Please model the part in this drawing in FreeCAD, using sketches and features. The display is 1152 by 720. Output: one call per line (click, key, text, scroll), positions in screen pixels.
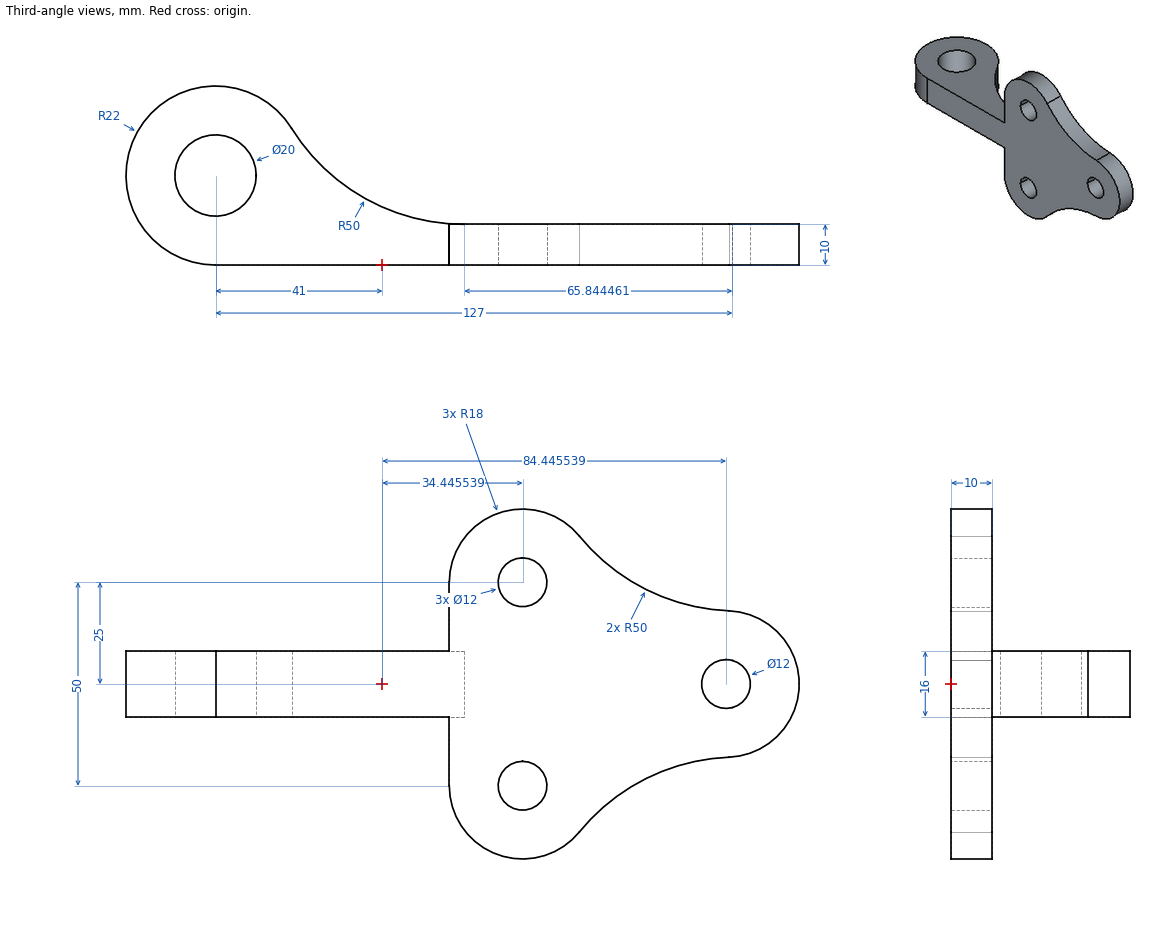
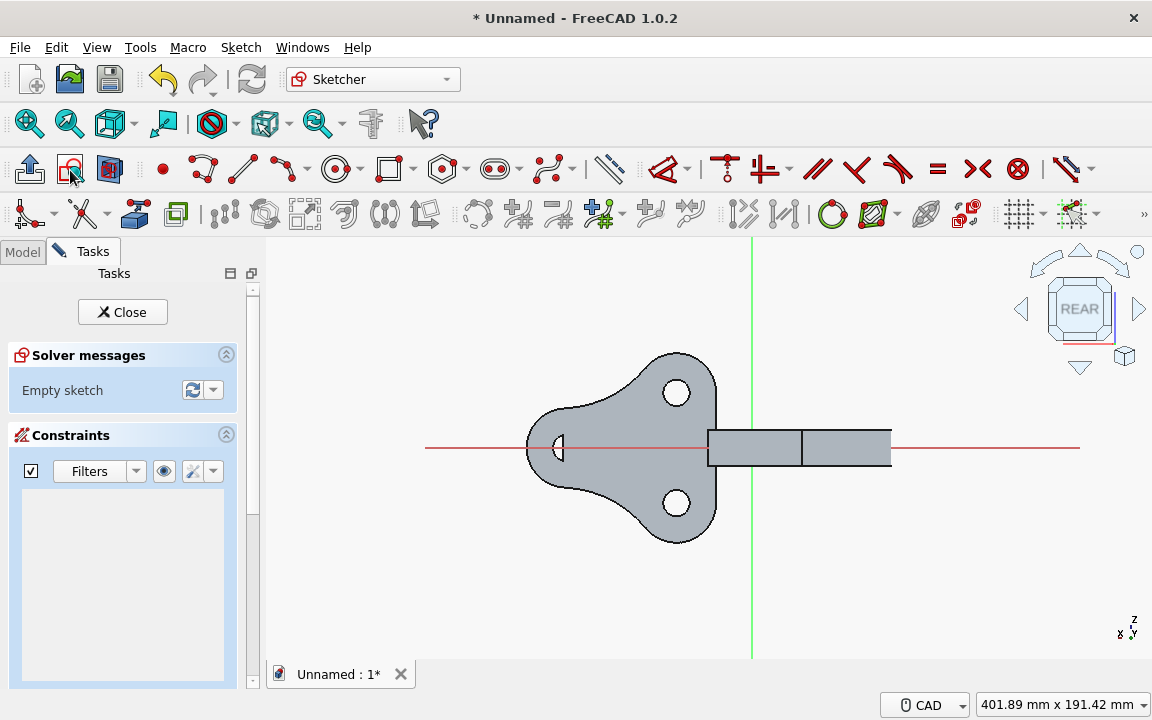
scroll(557, 448, up, 11)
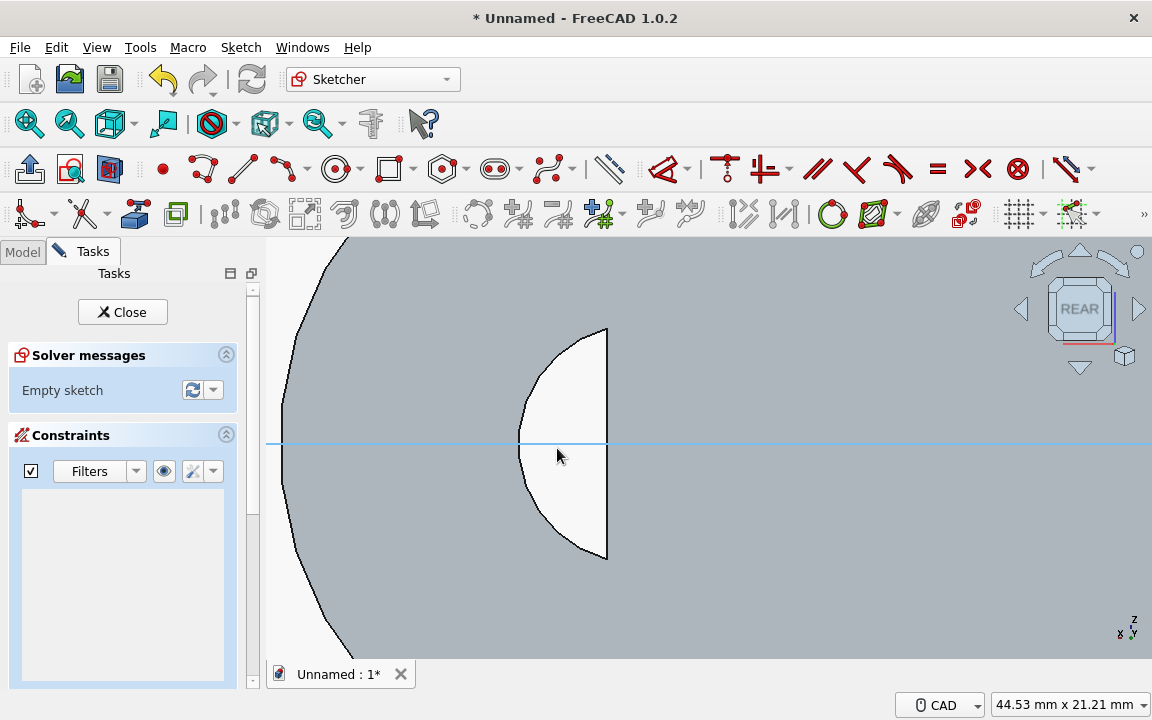
click(336, 170)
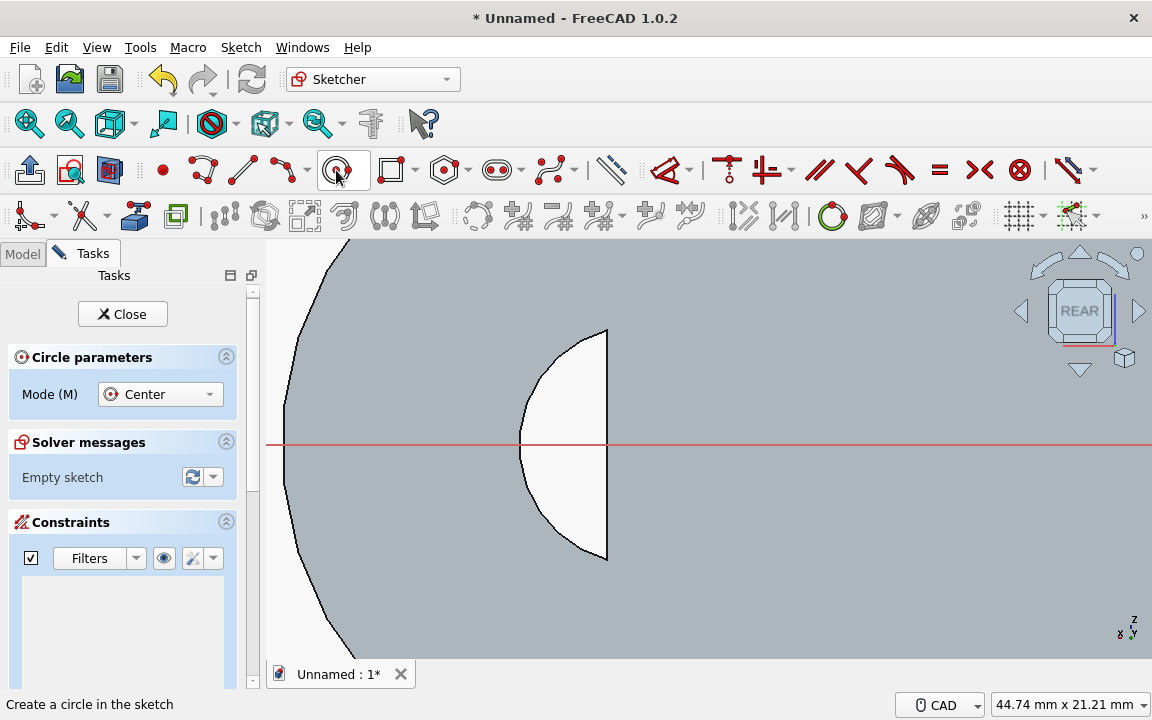
click(638, 445)
click(722, 361)
key(Escape)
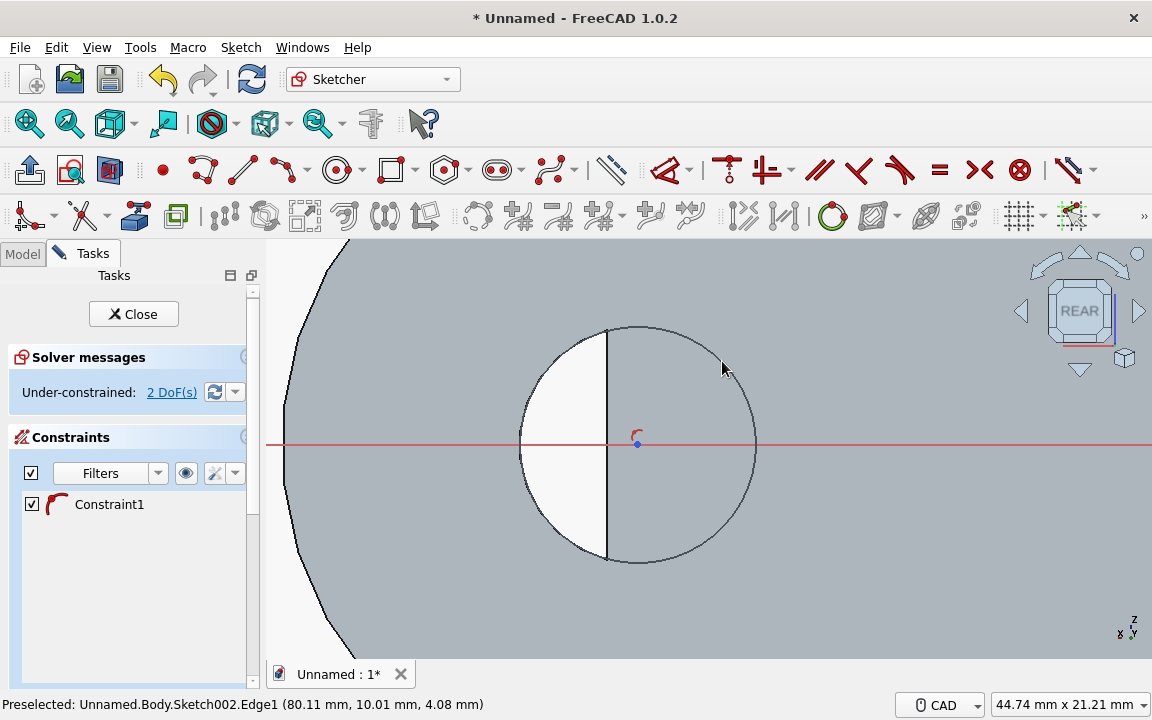
key(d)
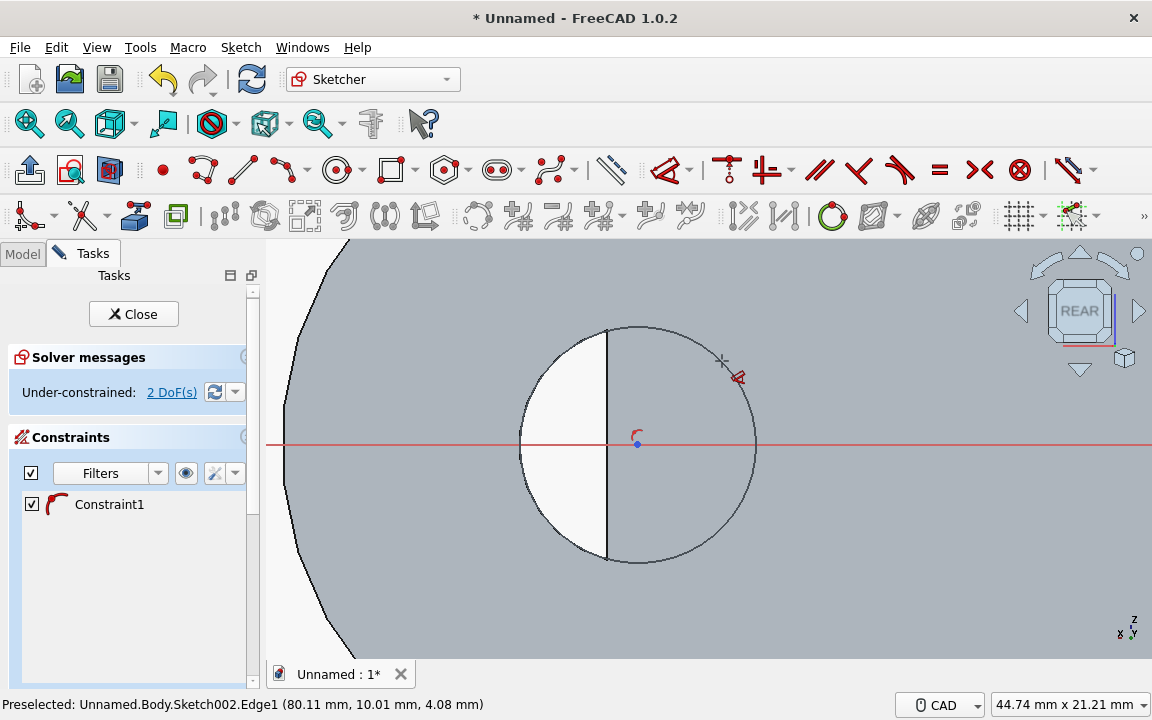
click(721, 361)
click(743, 338)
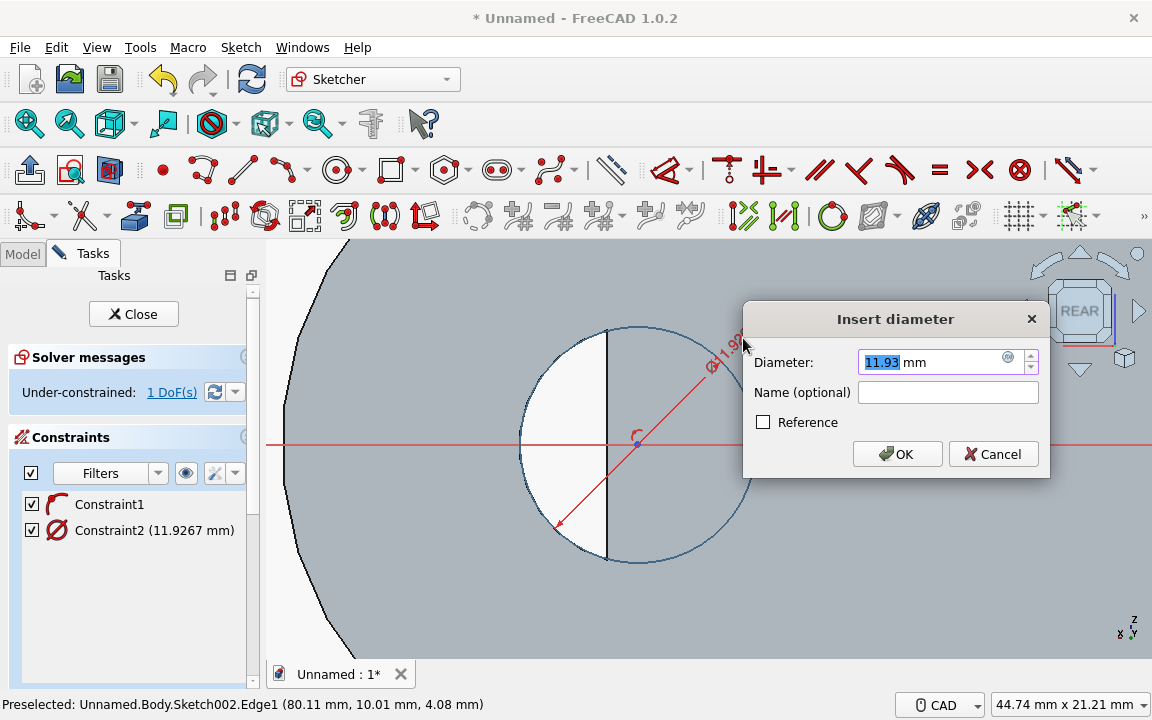
text(12)
key(Return)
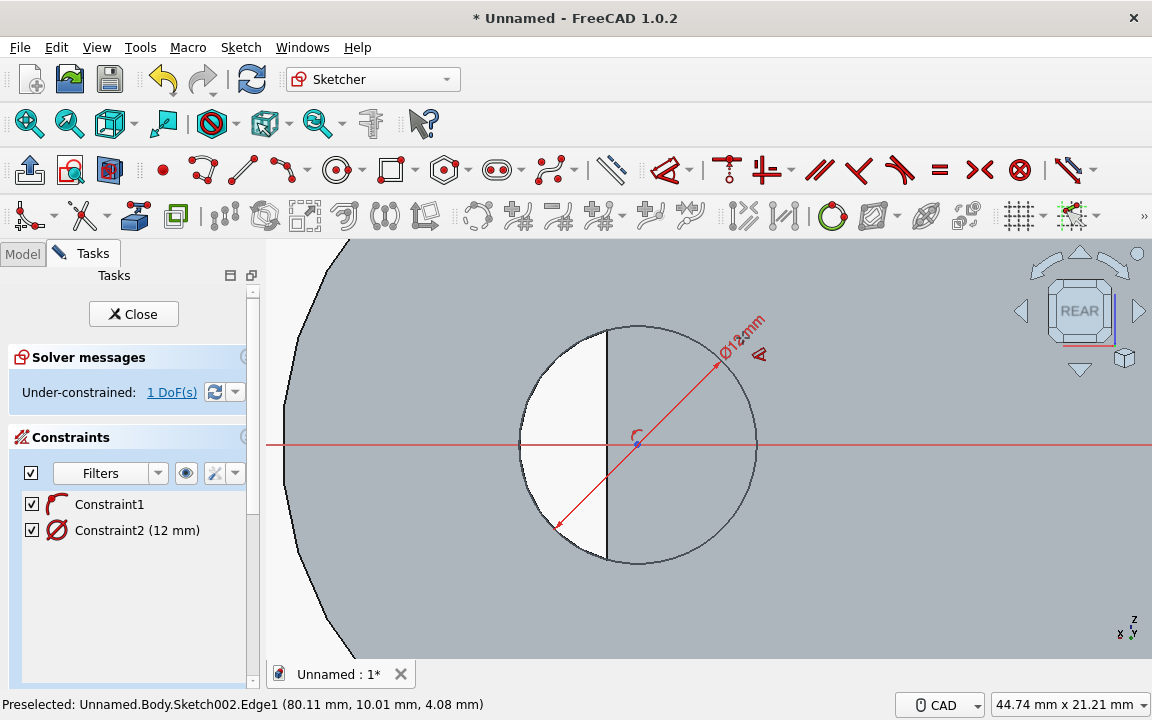
click(638, 445)
click(813, 479)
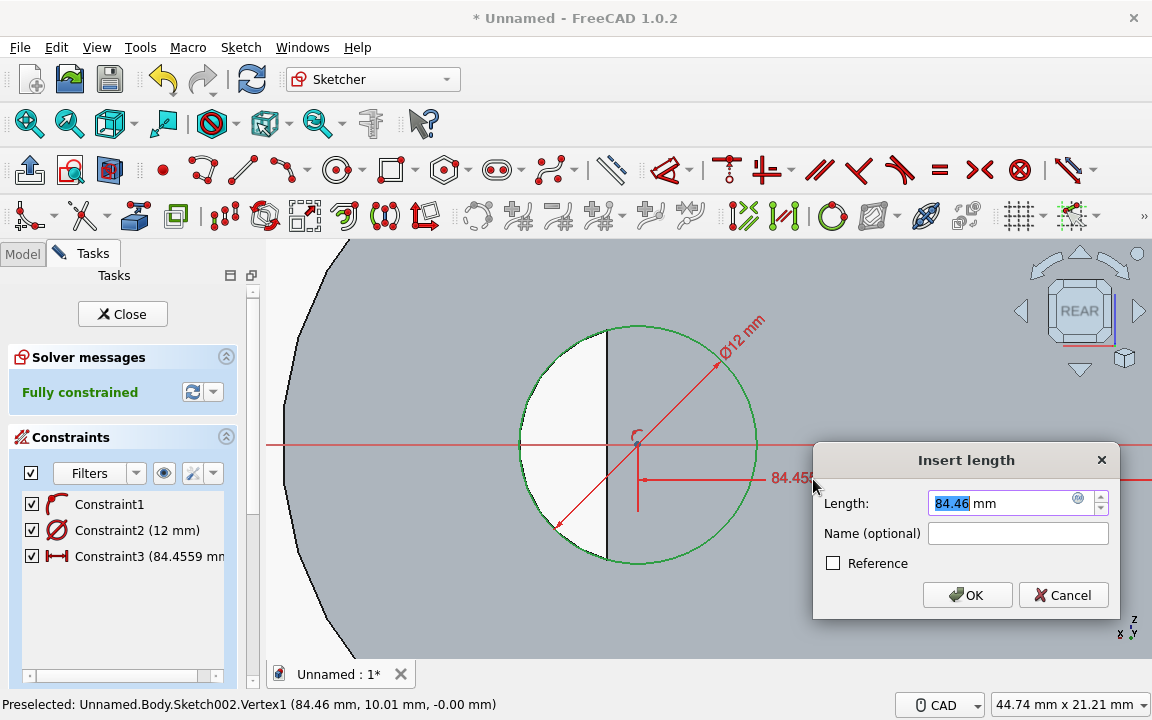
text(84.445539)
key(Return)
key(Escape)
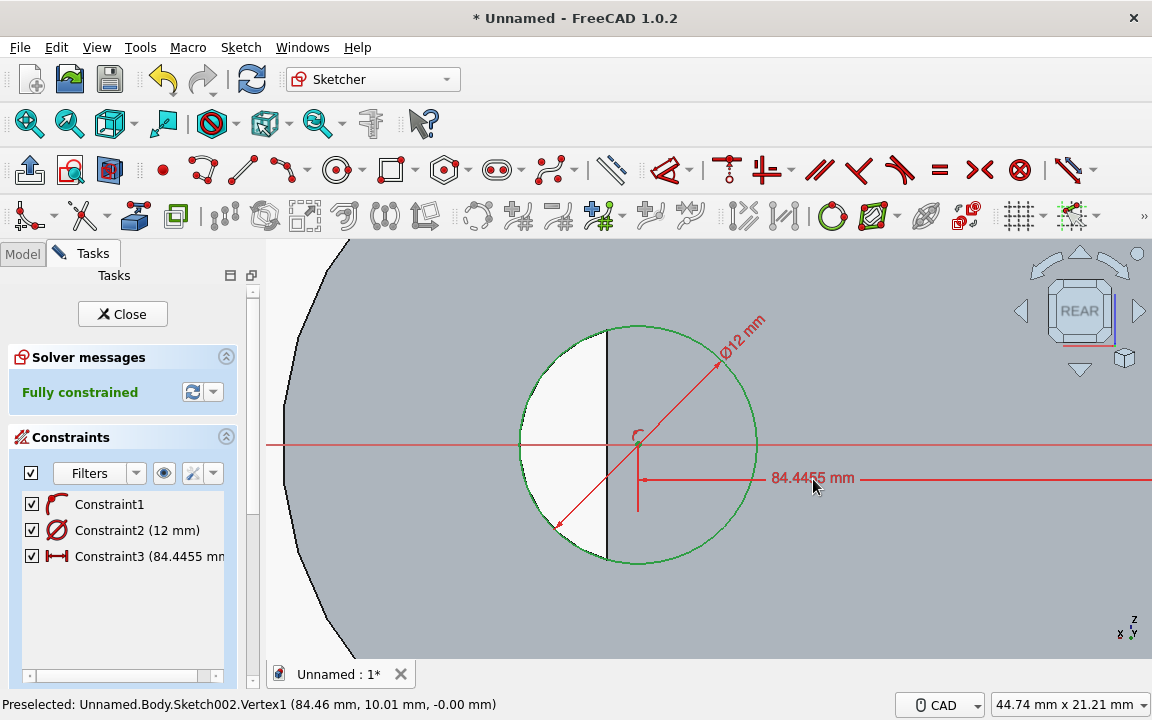
click(123, 314)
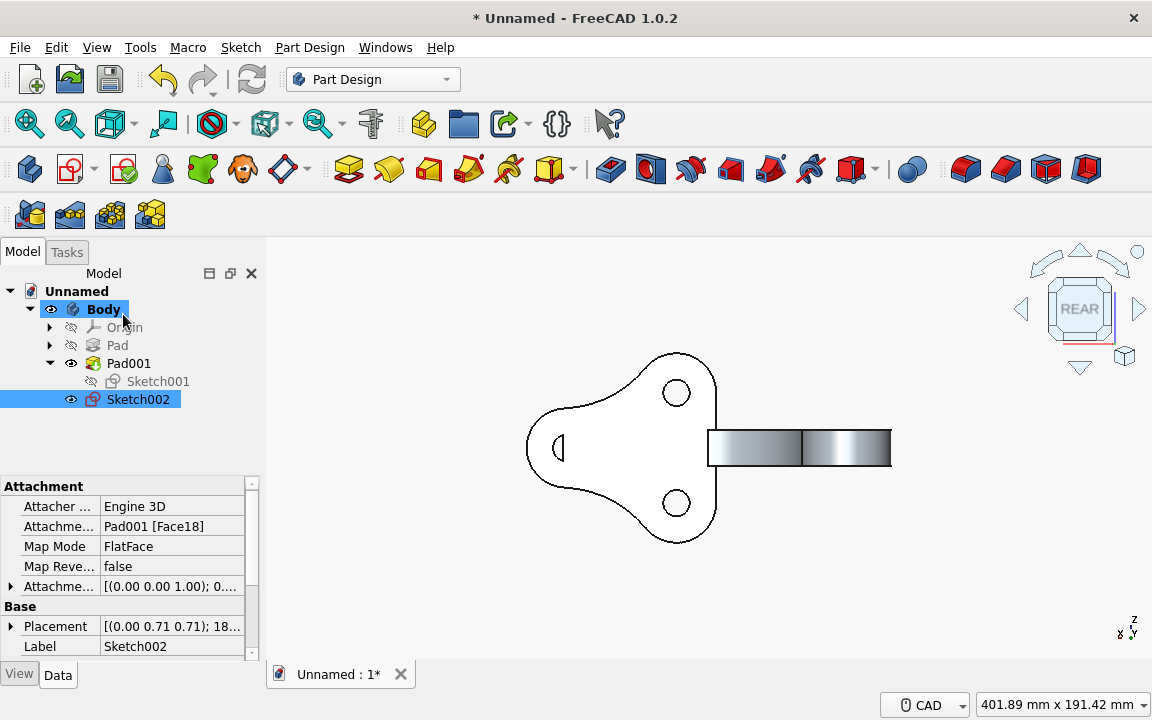
click(612, 170)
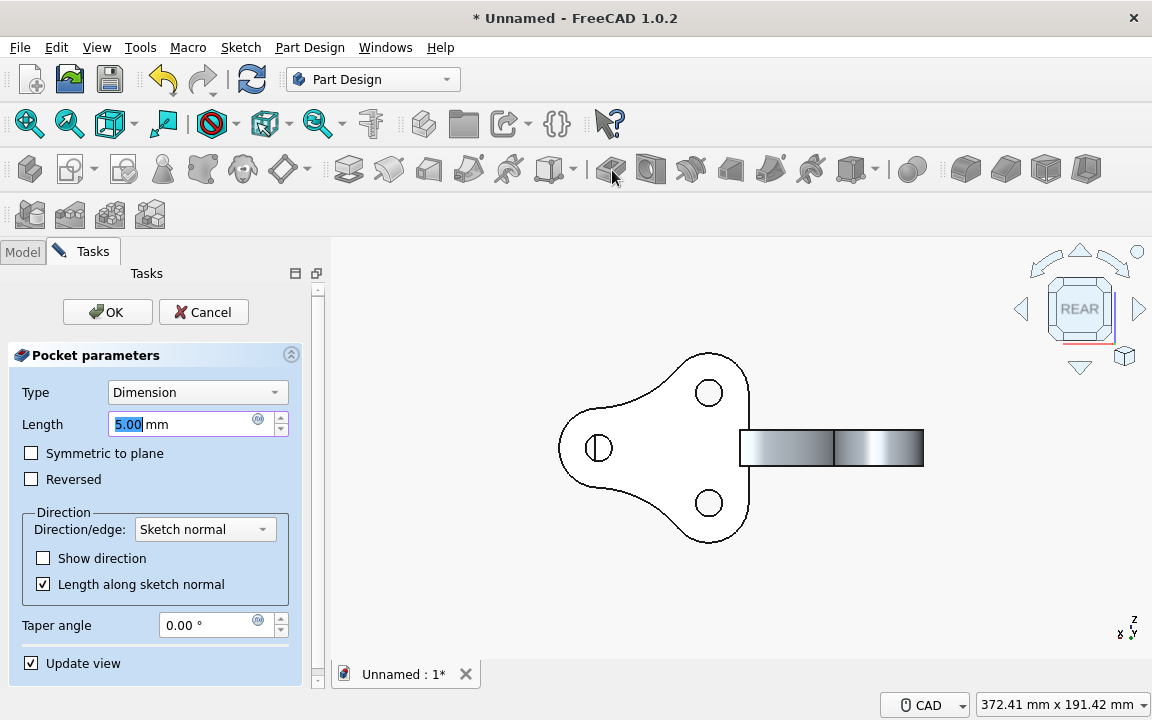
click(198, 392)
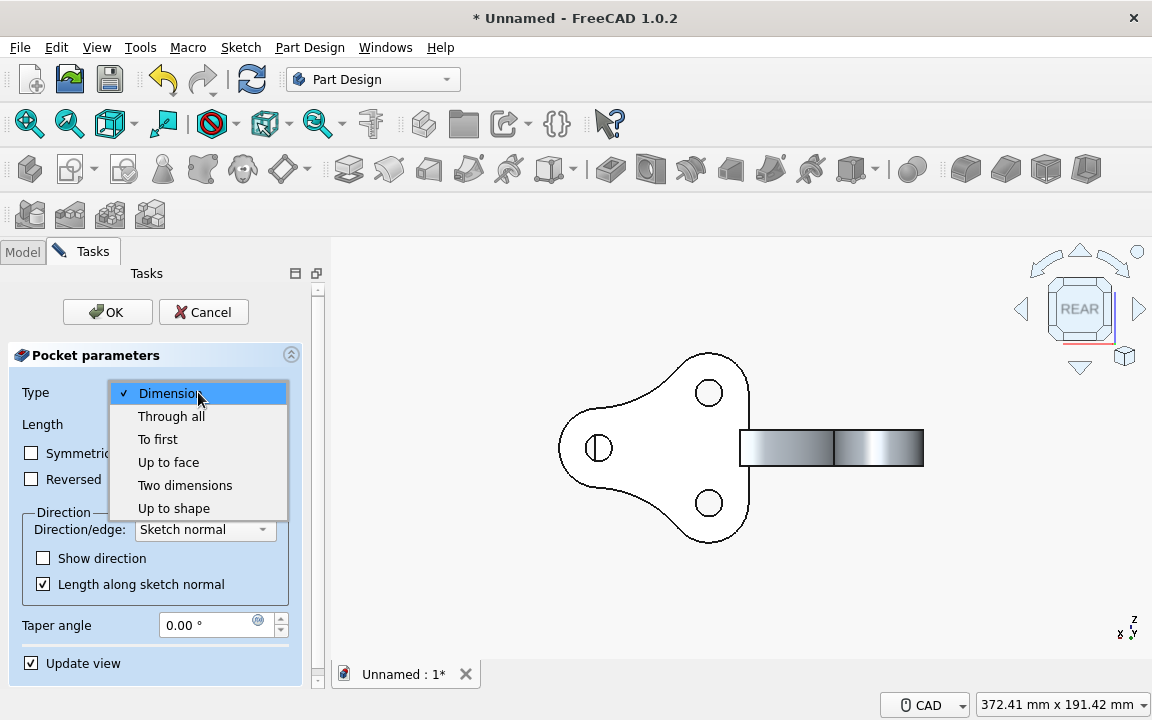
click(198, 416)